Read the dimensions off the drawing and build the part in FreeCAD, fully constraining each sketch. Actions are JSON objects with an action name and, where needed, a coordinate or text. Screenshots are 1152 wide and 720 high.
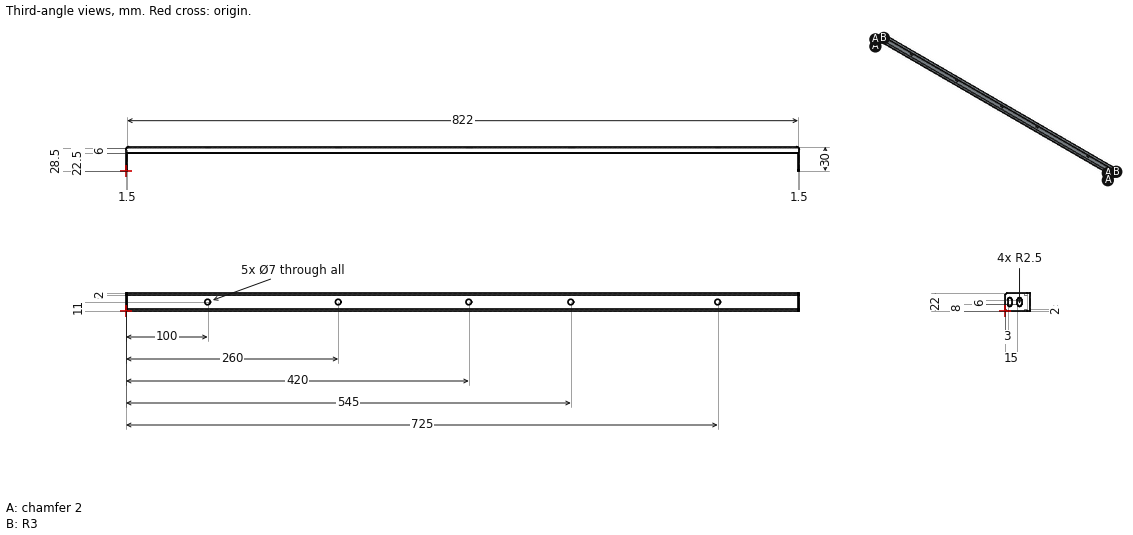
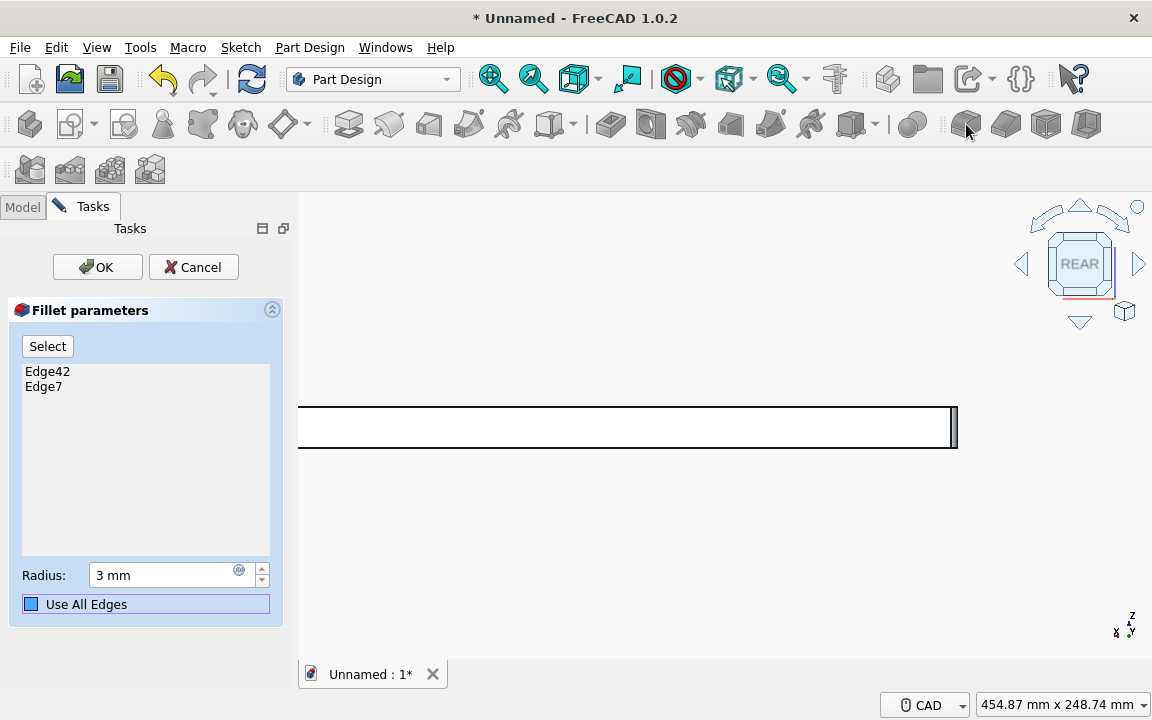
{"action": "left_click", "coordinate": [98, 267]}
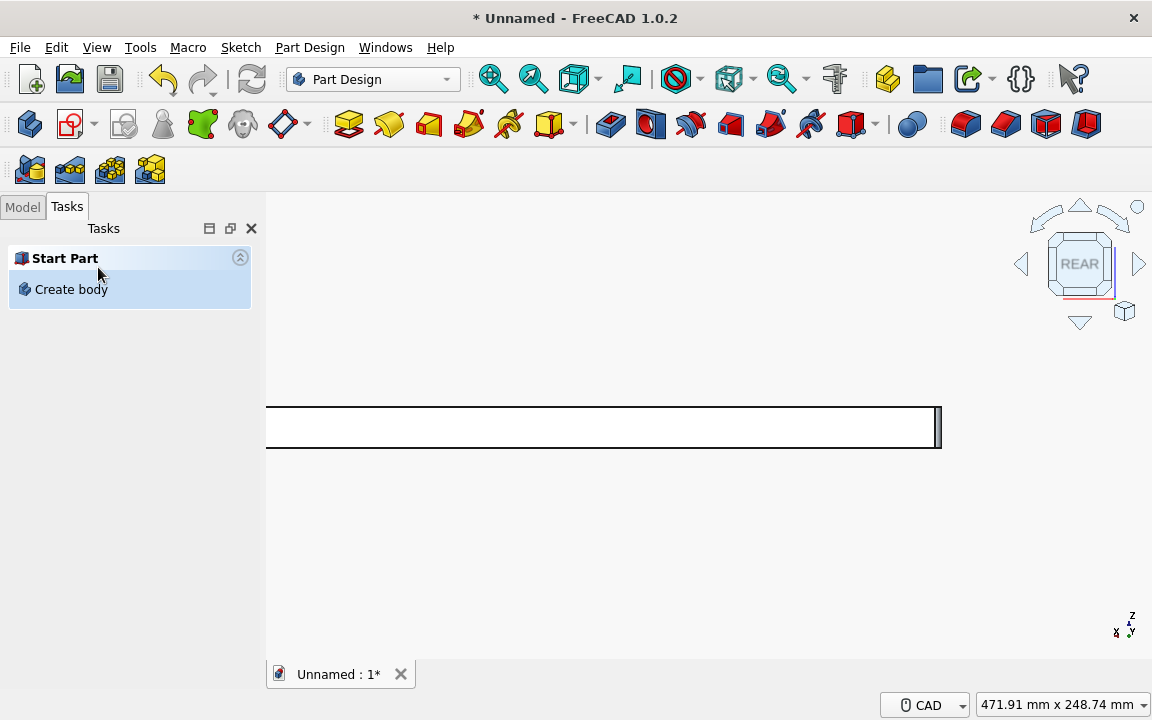
{"action": "left_click", "coordinate": [494, 80]}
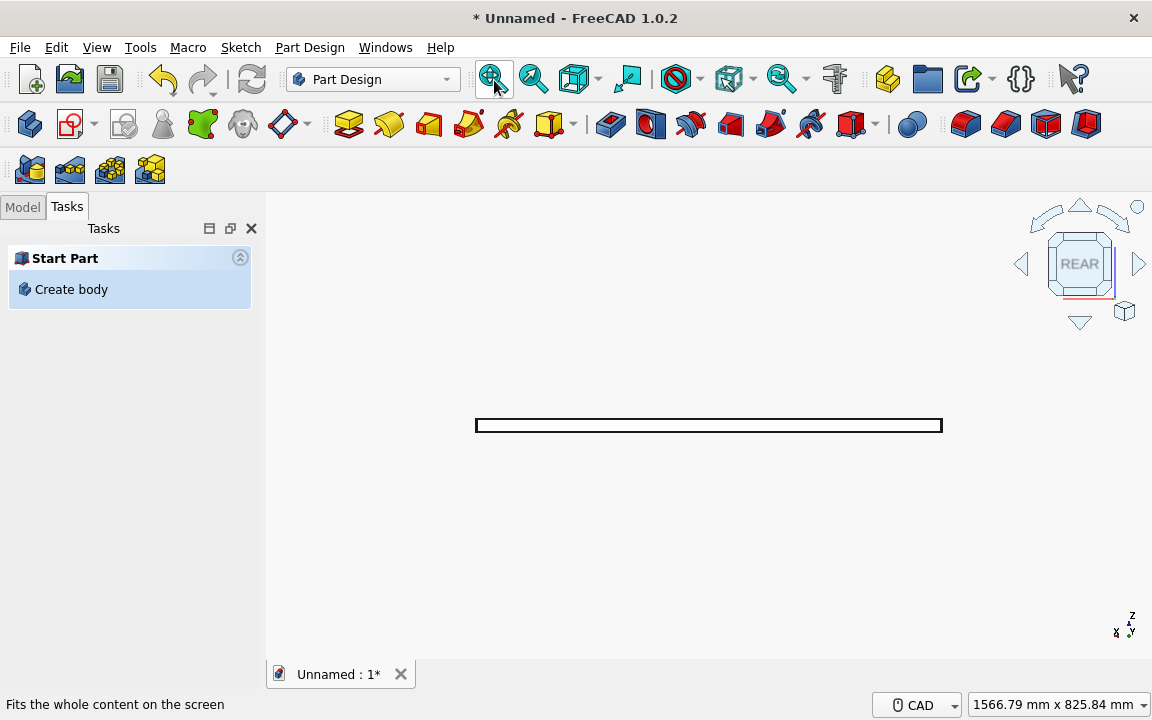
{"action": "key", "text": "0"}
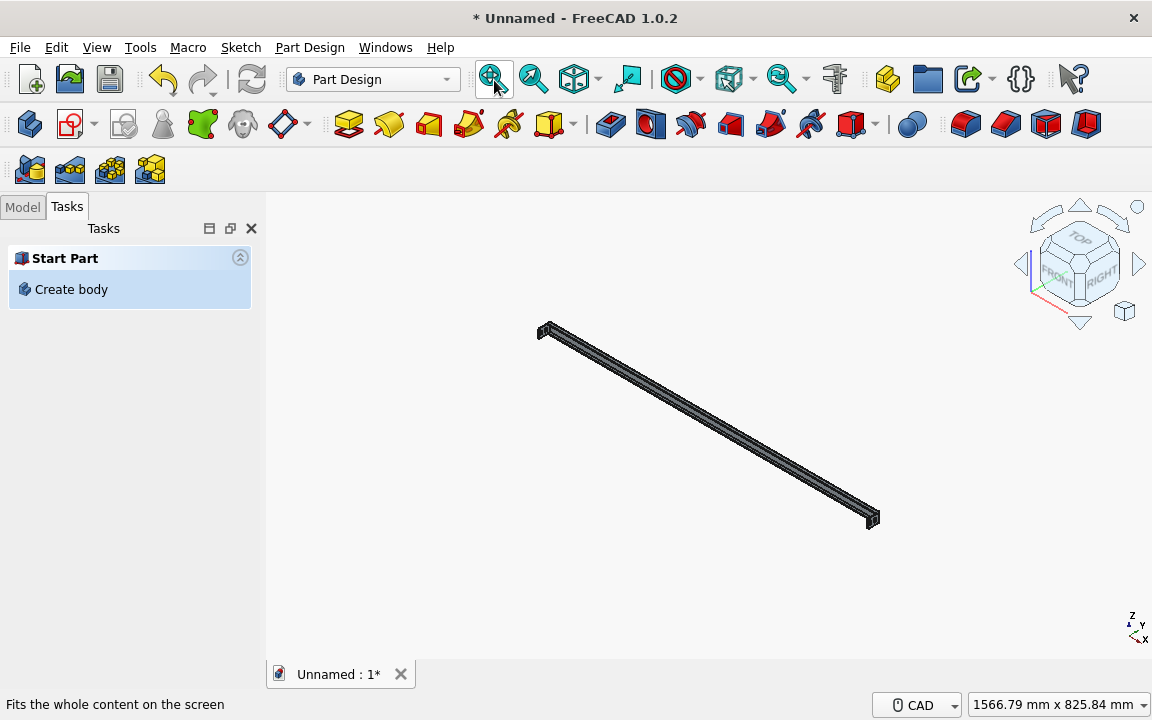
{"action": "left_click", "coordinate": [494, 80]}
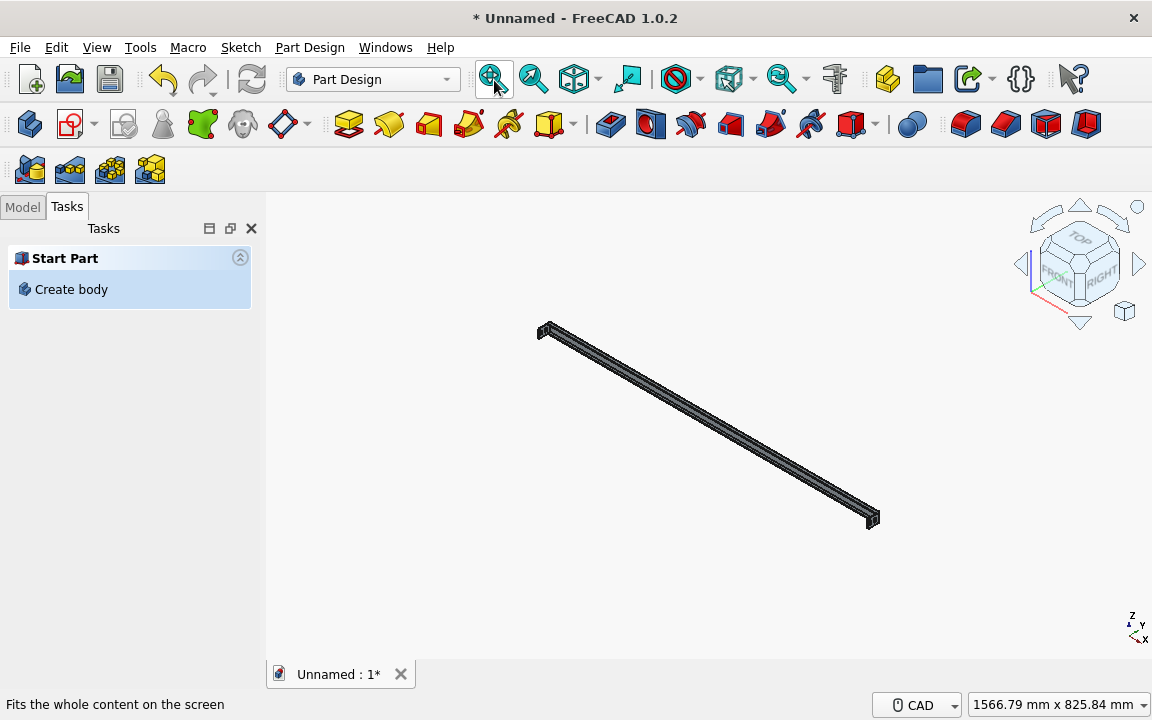
{"action": "scroll", "coordinate": [855, 503], "scroll_direction": "up", "scroll_amount": 5}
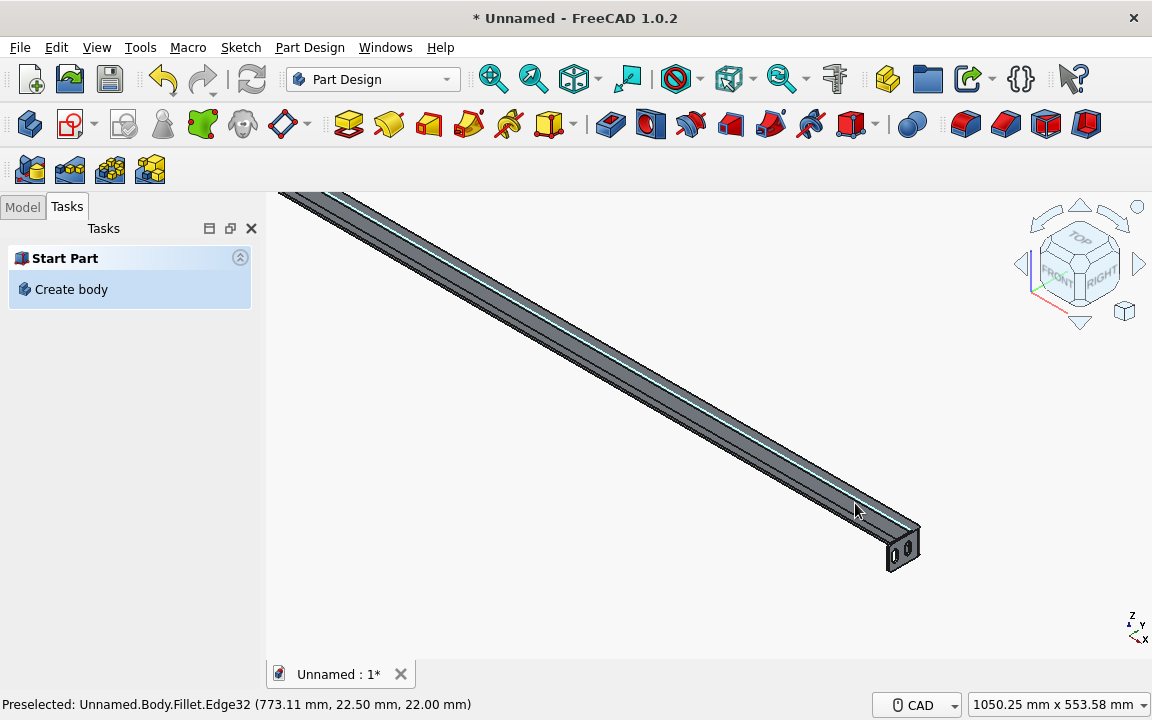
{"action": "left_click", "coordinate": [494, 80]}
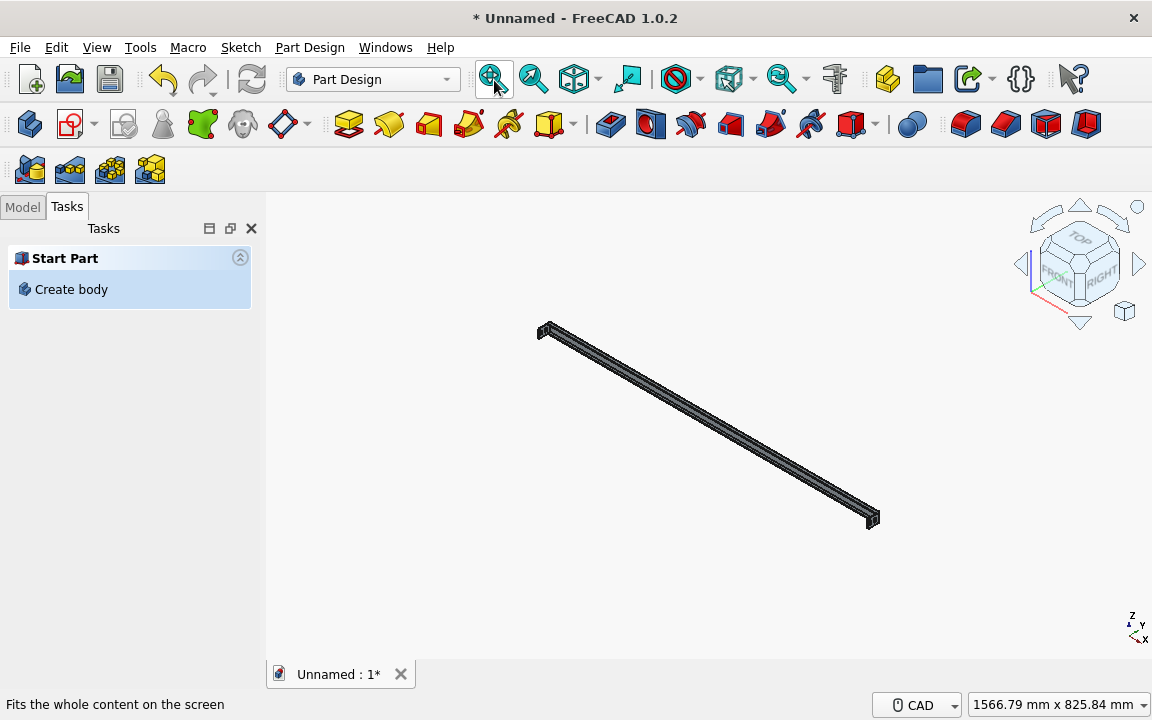
{"action": "key", "text": "1"}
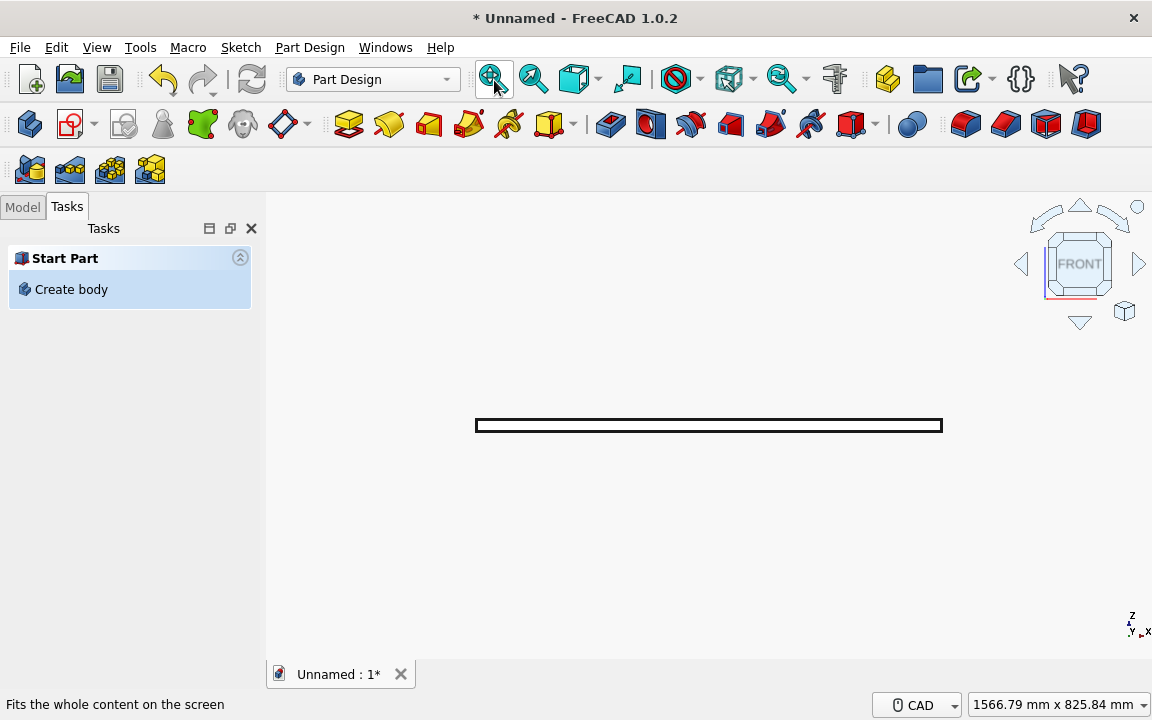
{"action": "scroll", "coordinate": [908, 424], "scroll_direction": "up", "scroll_amount": 5}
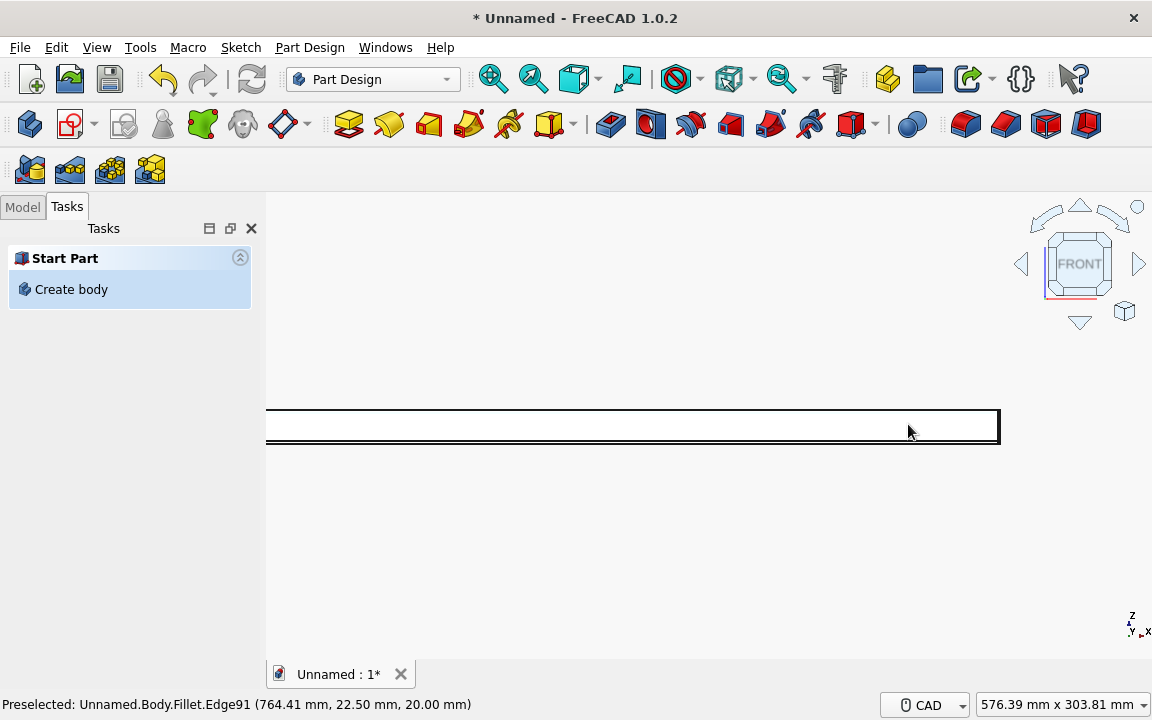
{"action": "left_click", "coordinate": [907, 426]}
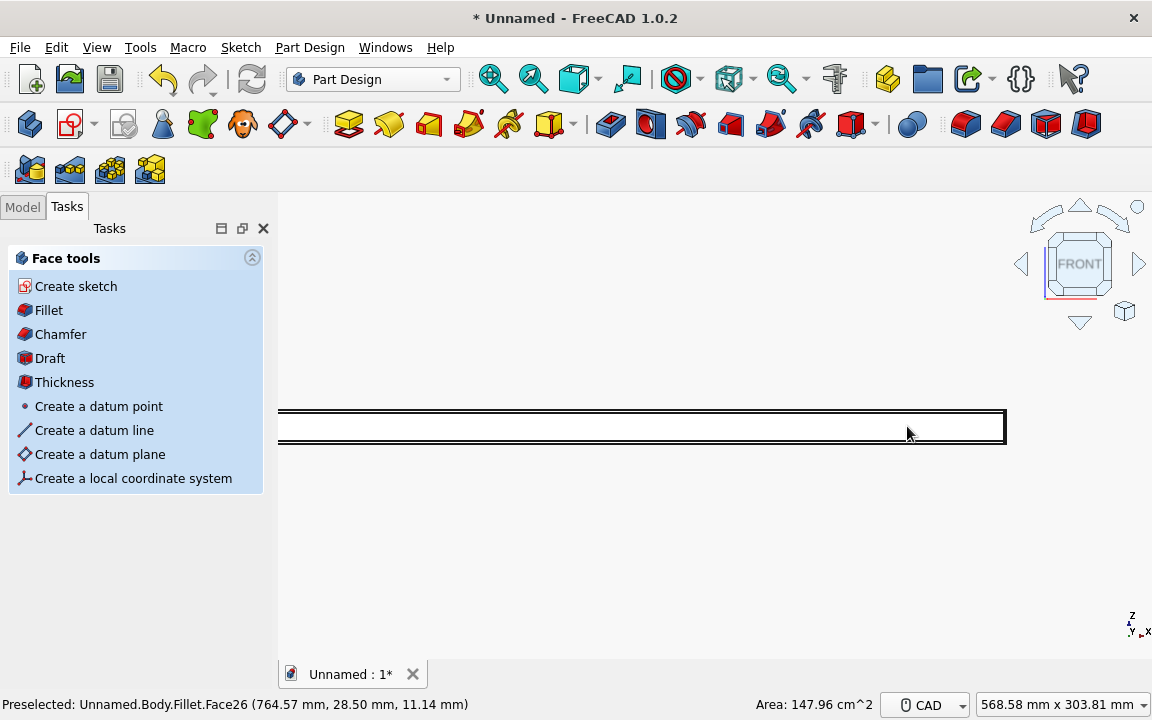
{"action": "left_click", "coordinate": [70, 124]}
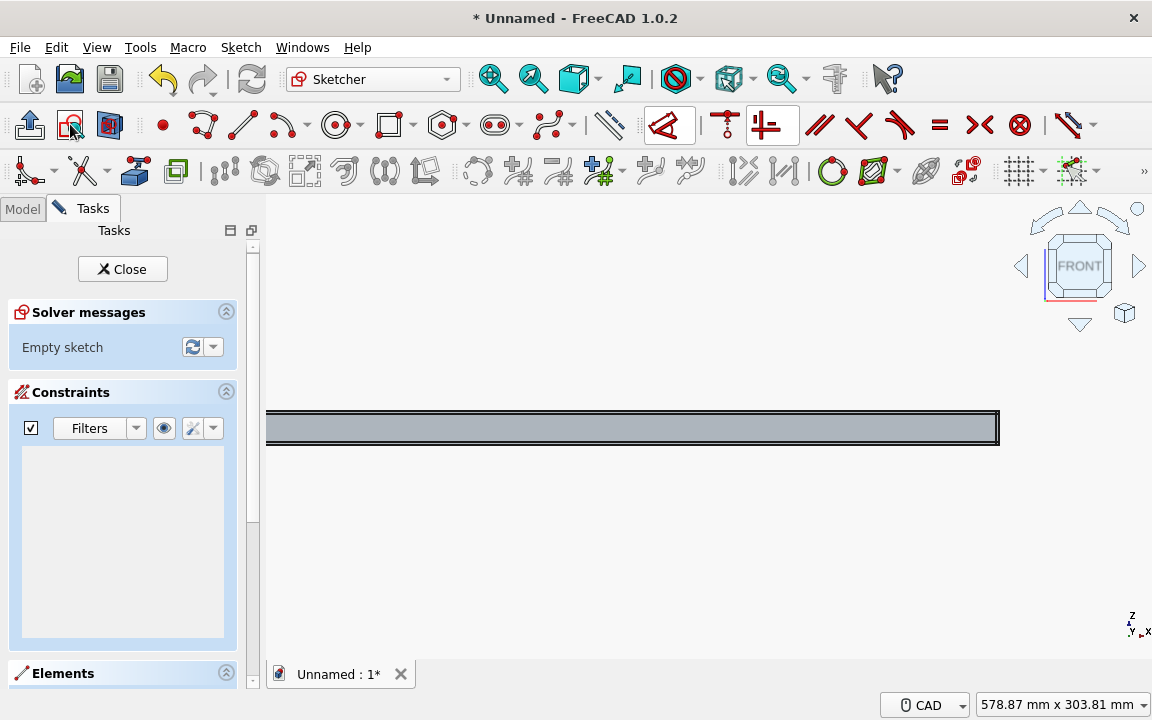
{"action": "scroll", "coordinate": [924, 420], "scroll_direction": "down", "scroll_amount": 4}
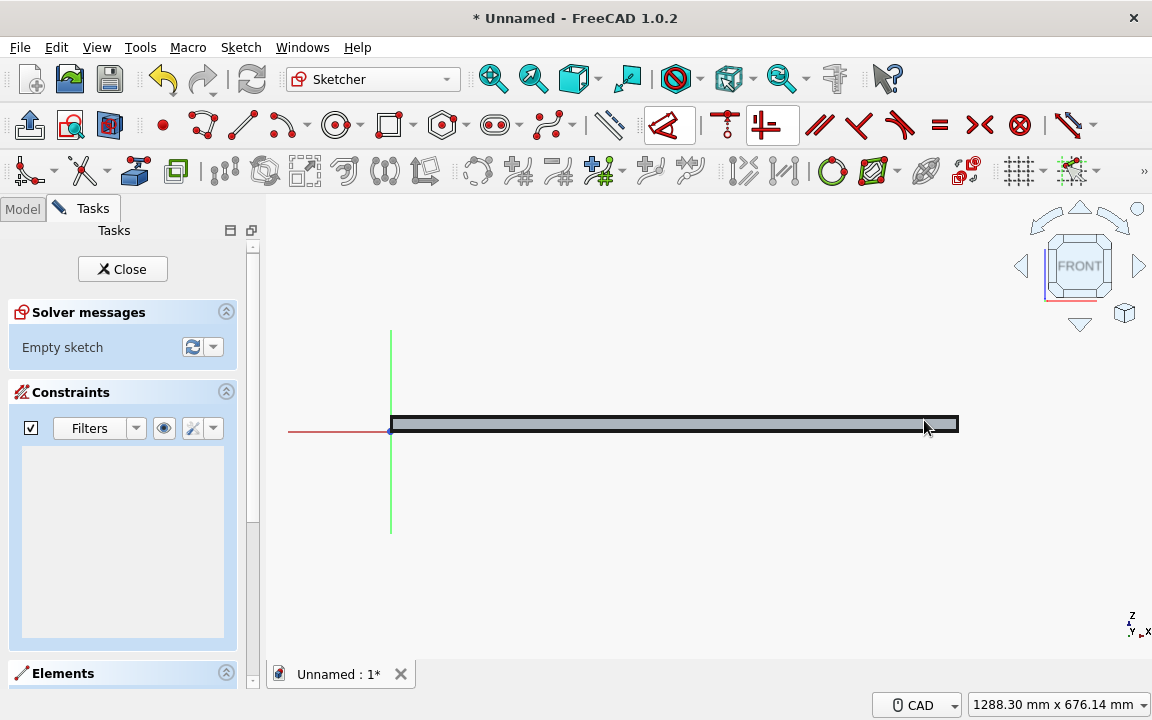
{"action": "left_click", "coordinate": [336, 126]}